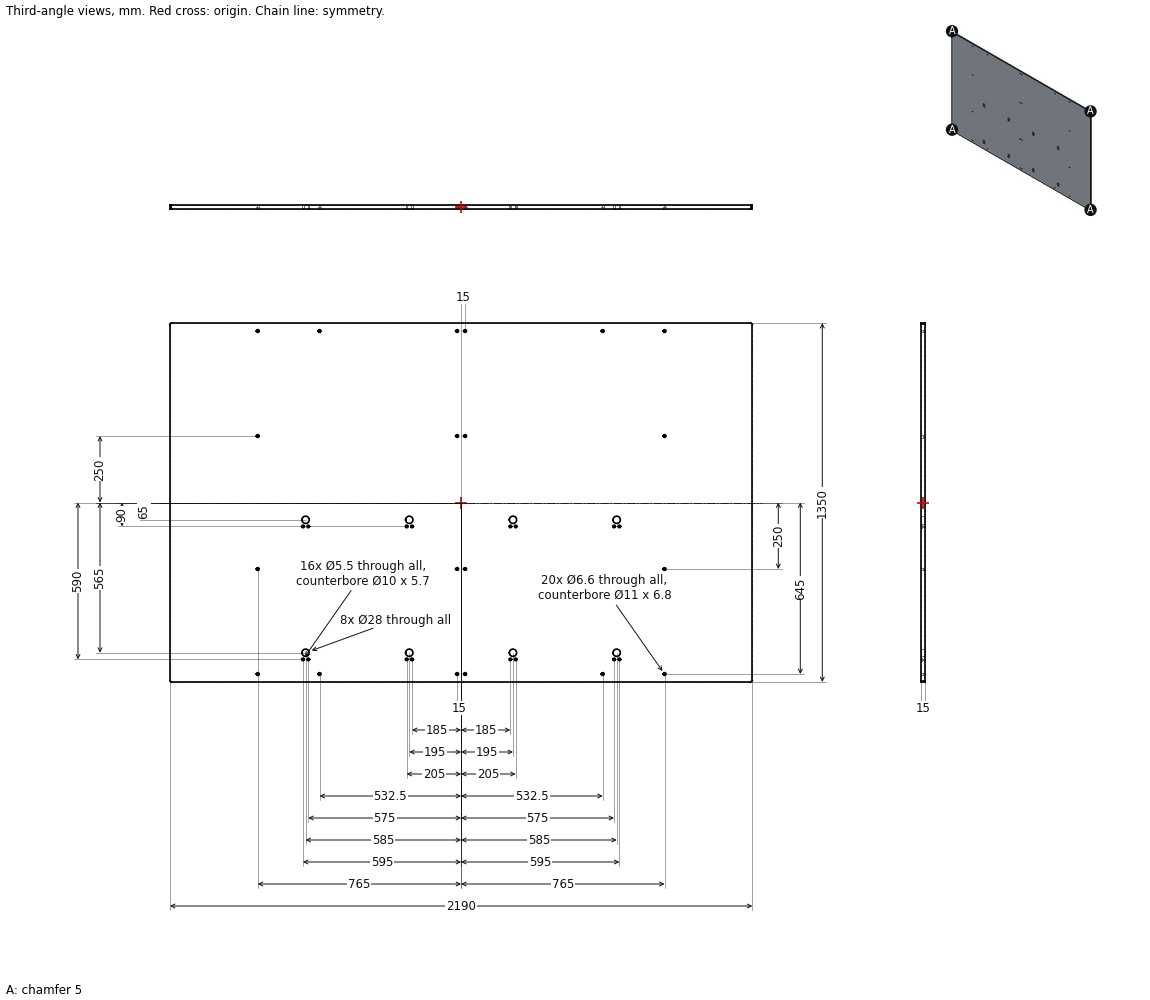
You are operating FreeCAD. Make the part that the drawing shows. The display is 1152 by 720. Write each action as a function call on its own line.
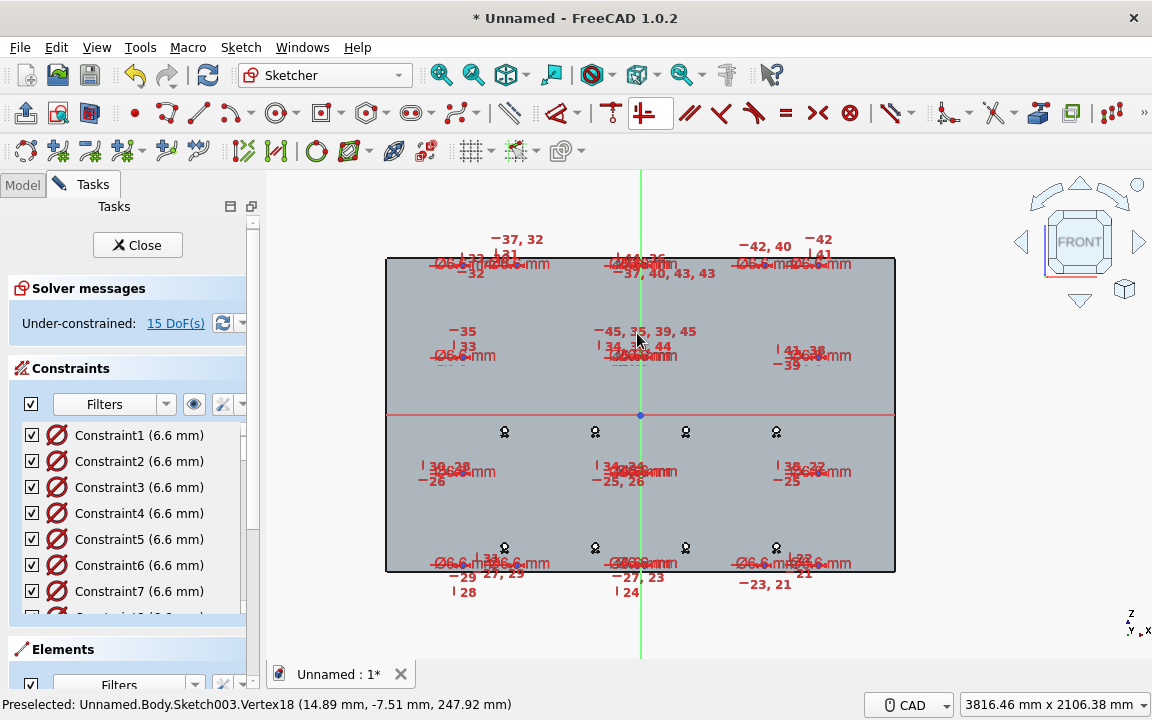
scroll(644, 473, up, 3)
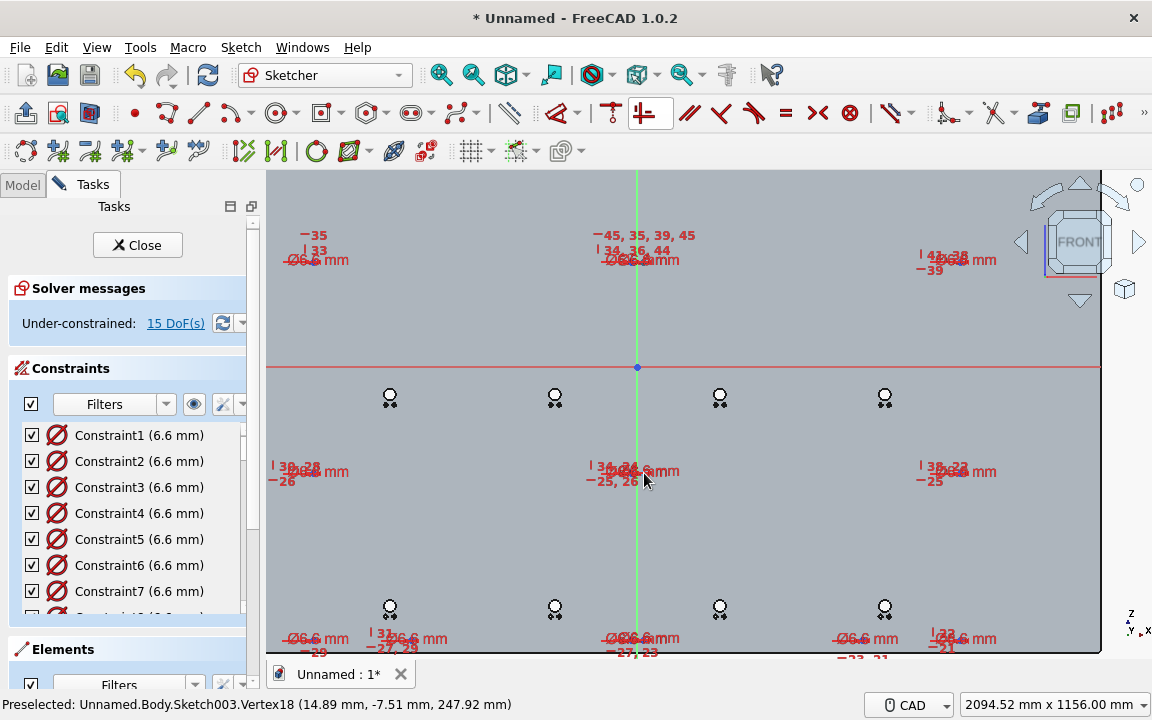
click(644, 473)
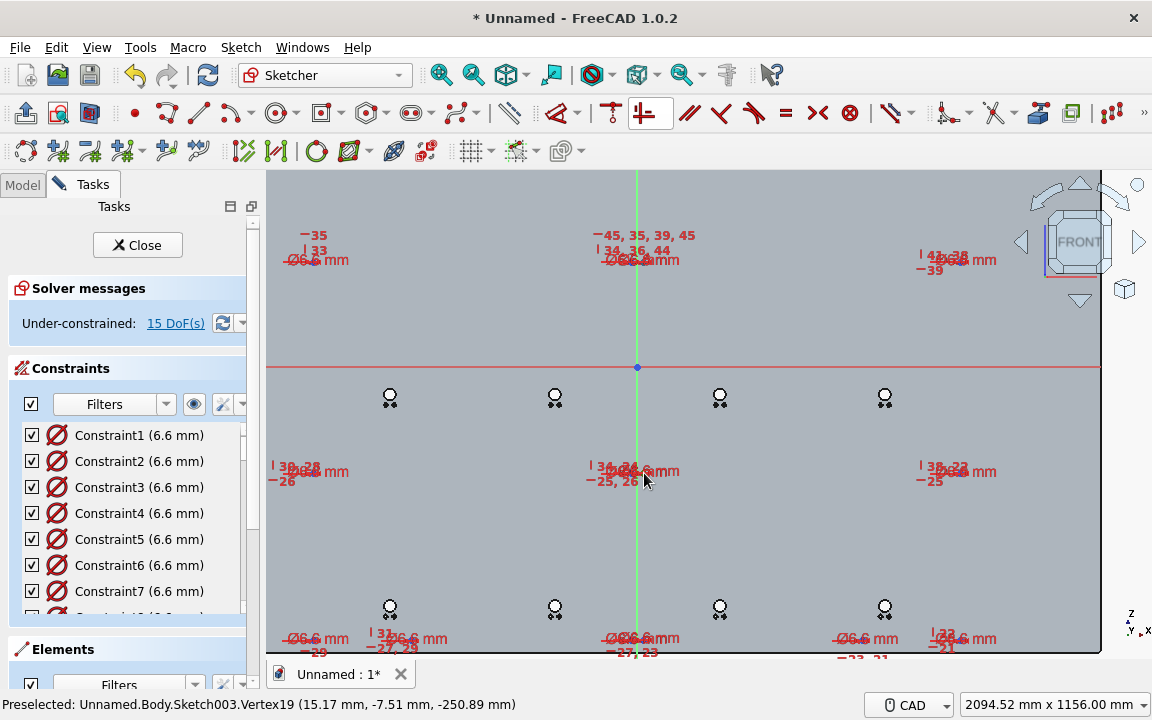
key(v)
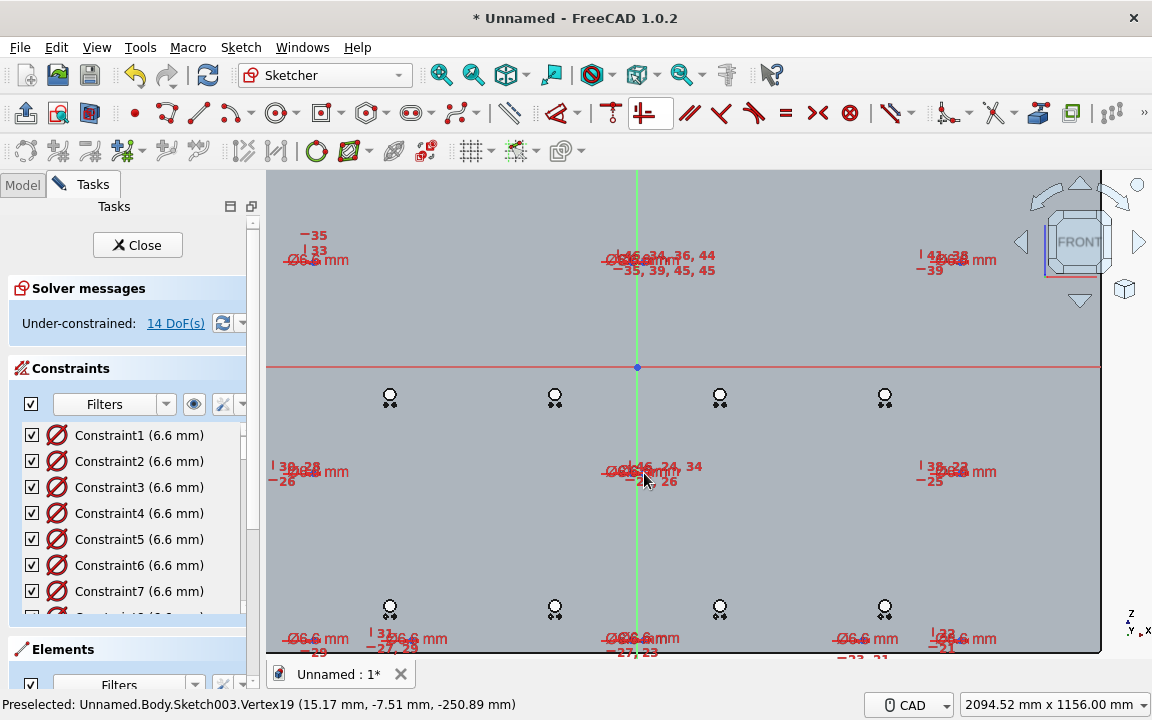
scroll(631, 474, up, 4)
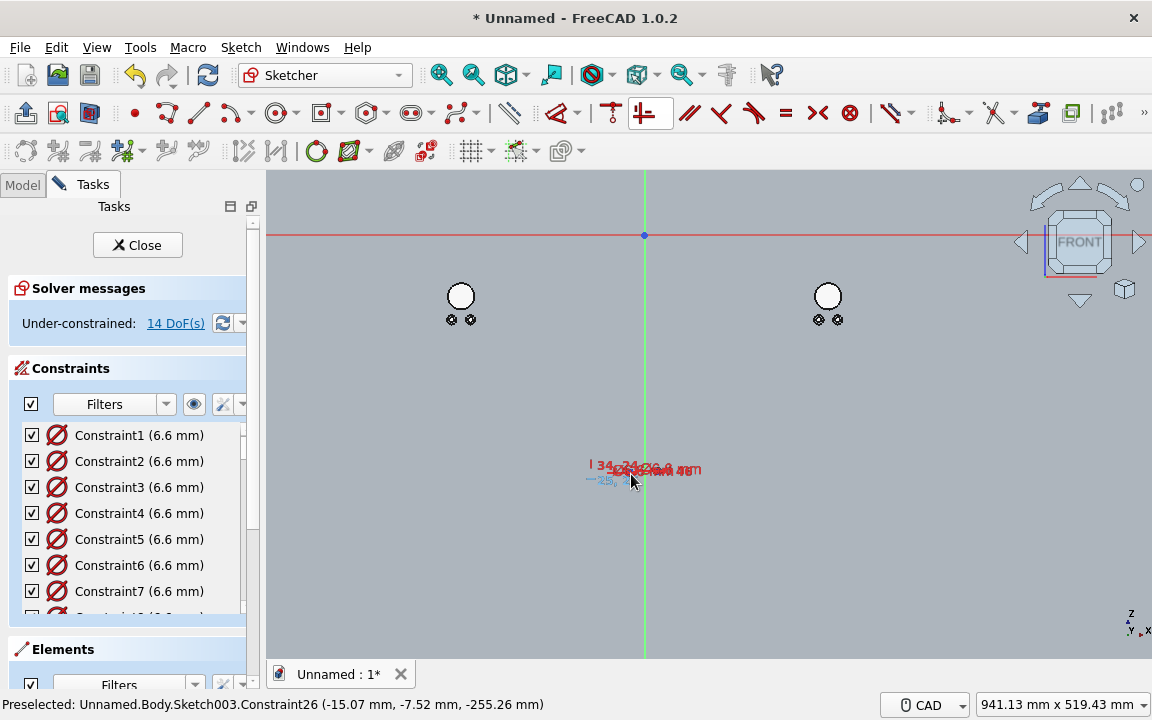
click(631, 473)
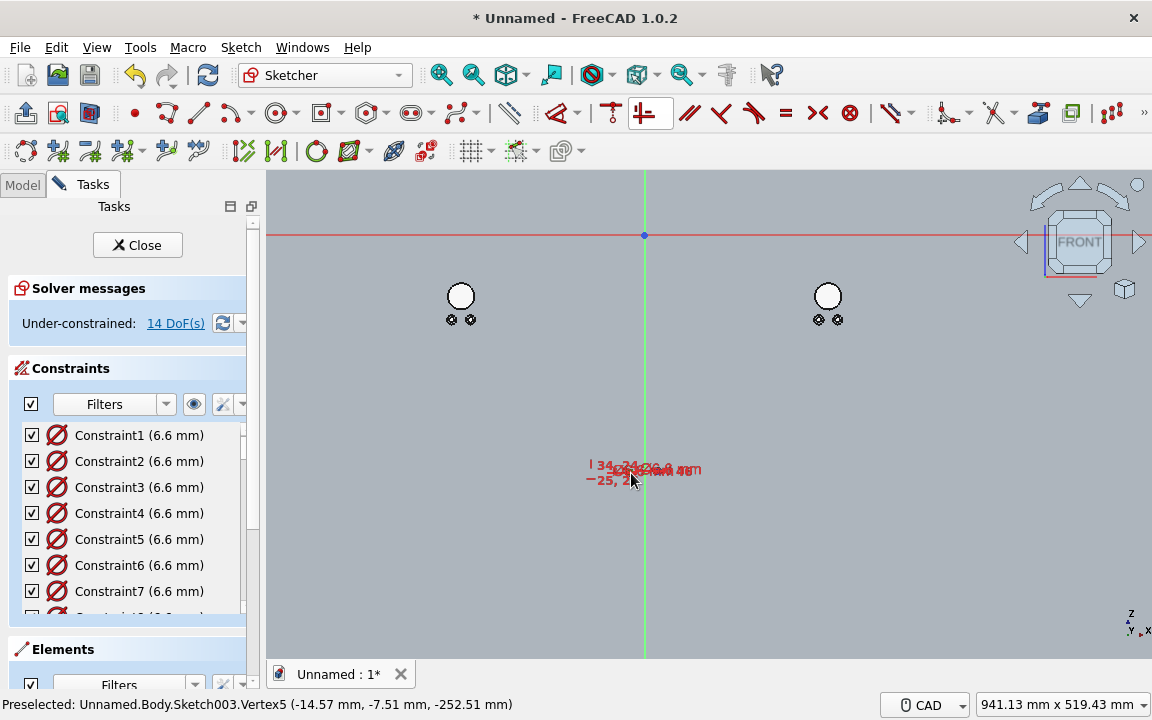
click(659, 471)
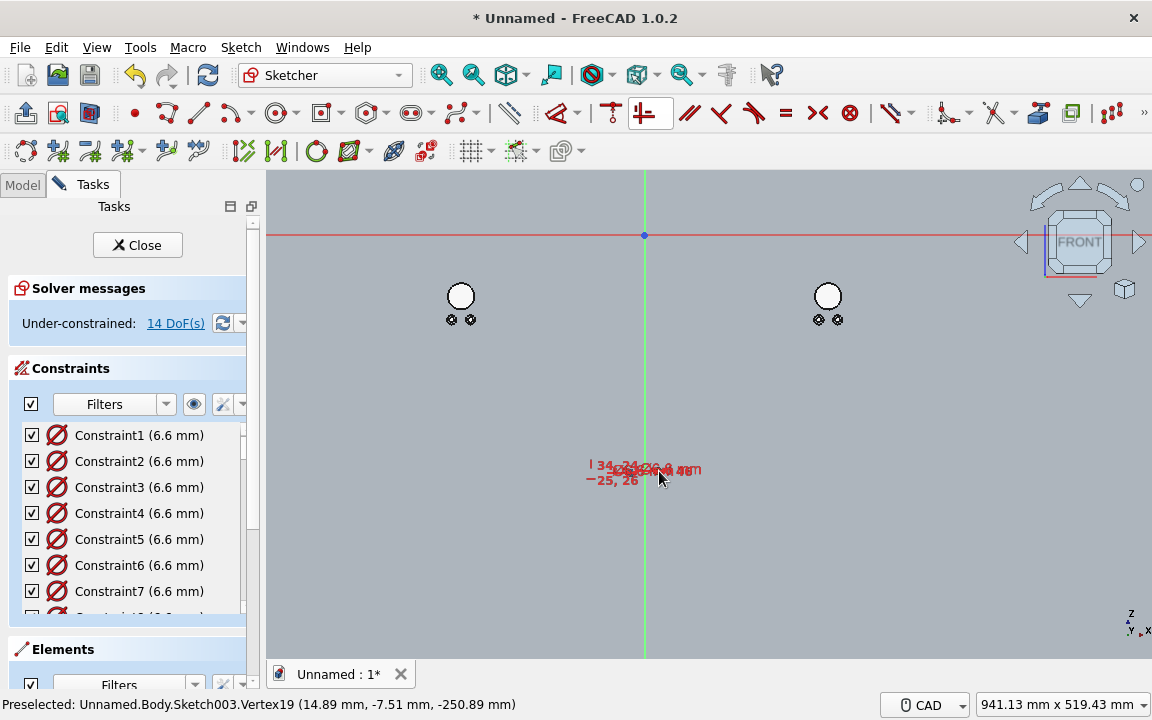
key(h)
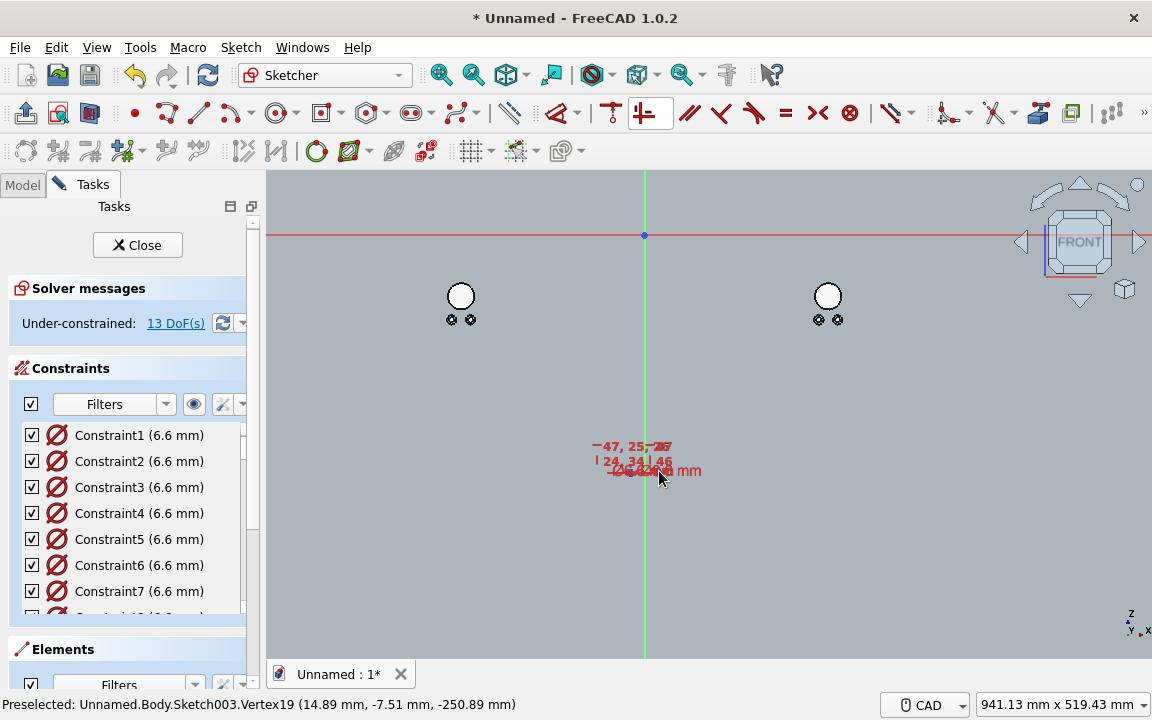
click(659, 473)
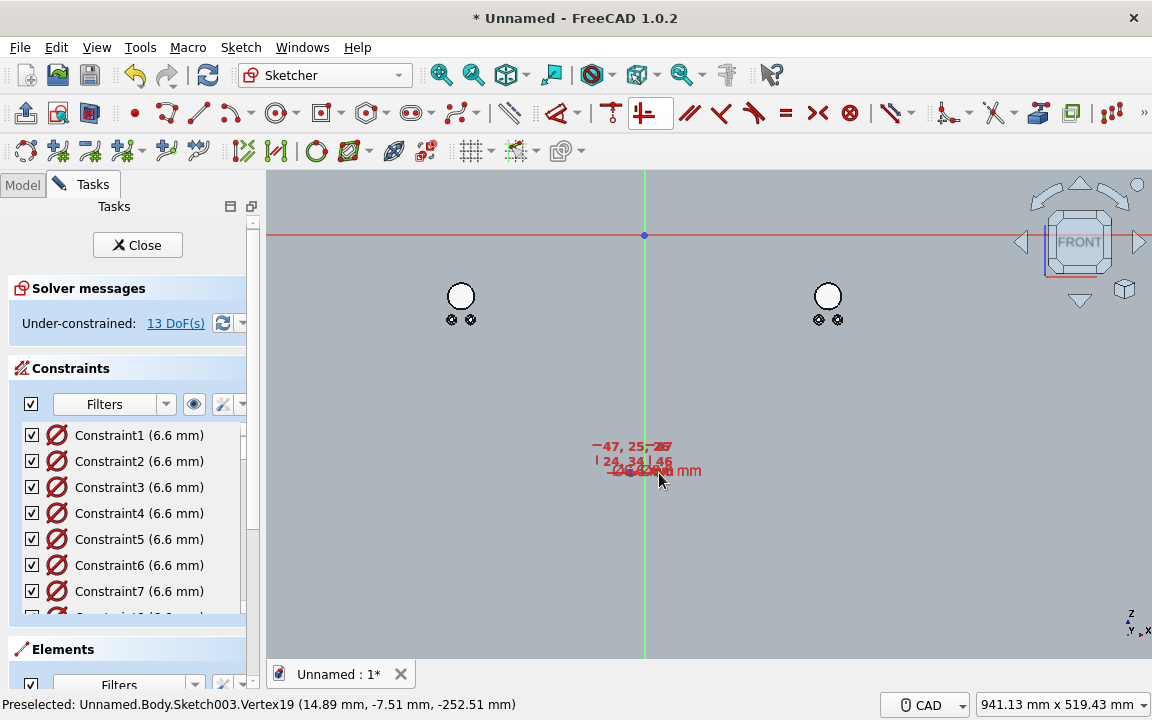
scroll(639, 473, down, 7)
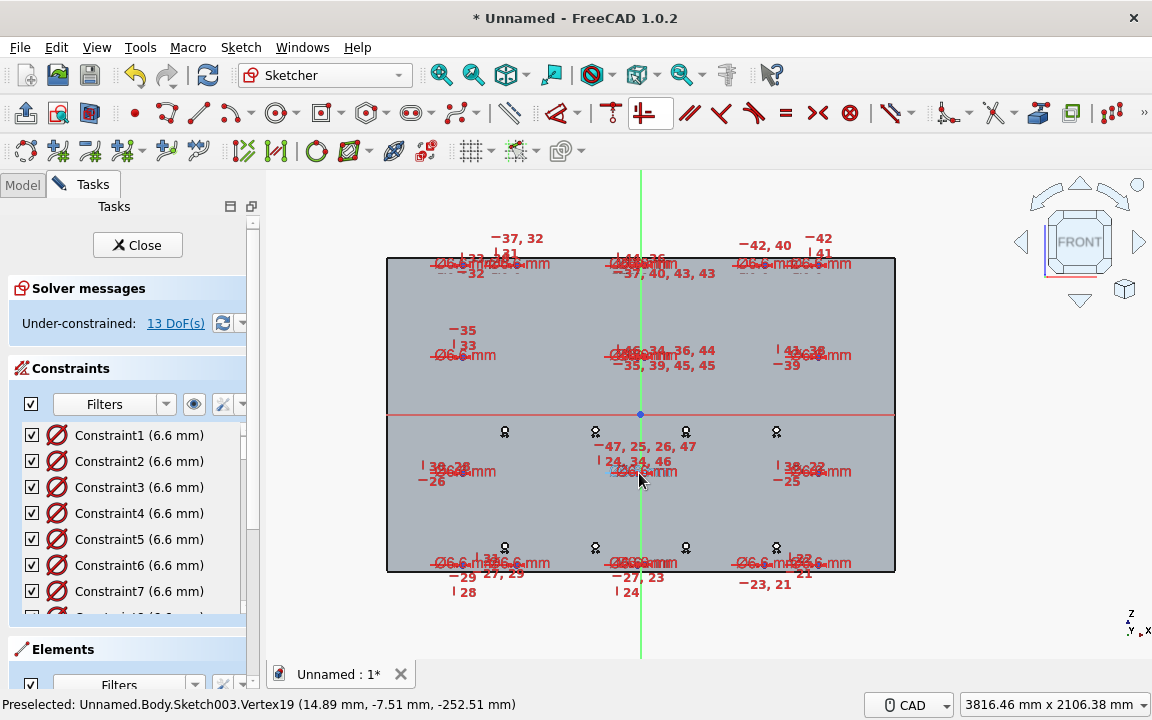
scroll(644, 565, up, 3)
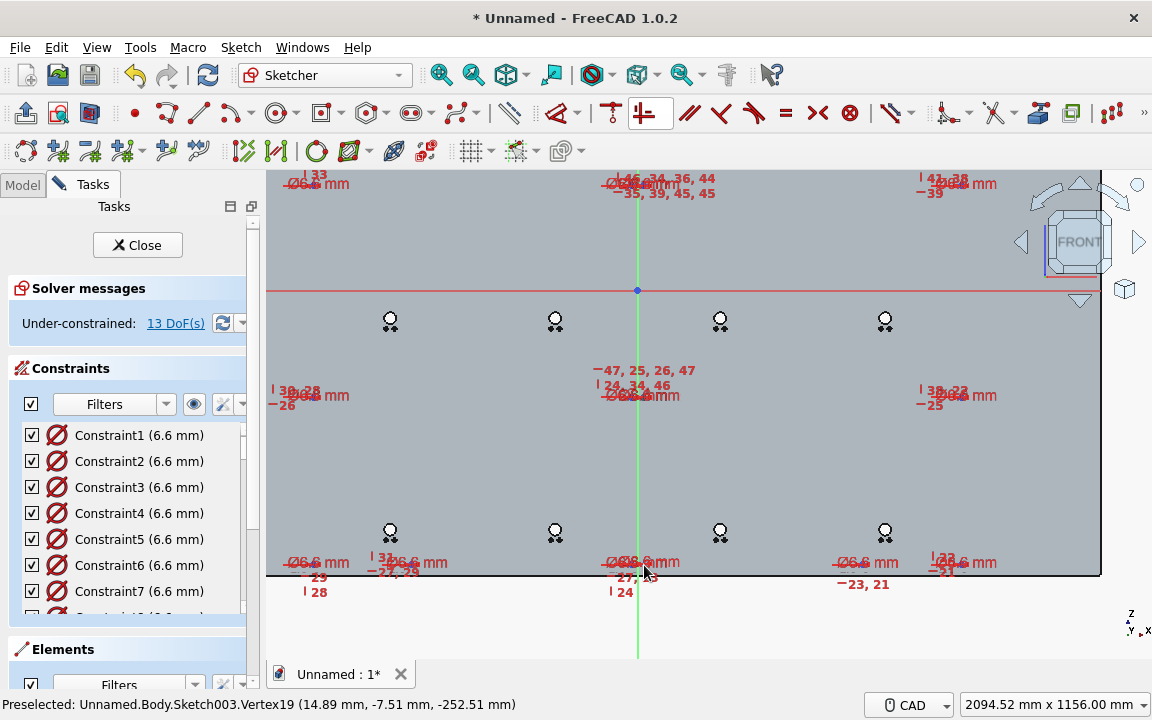
click(644, 564)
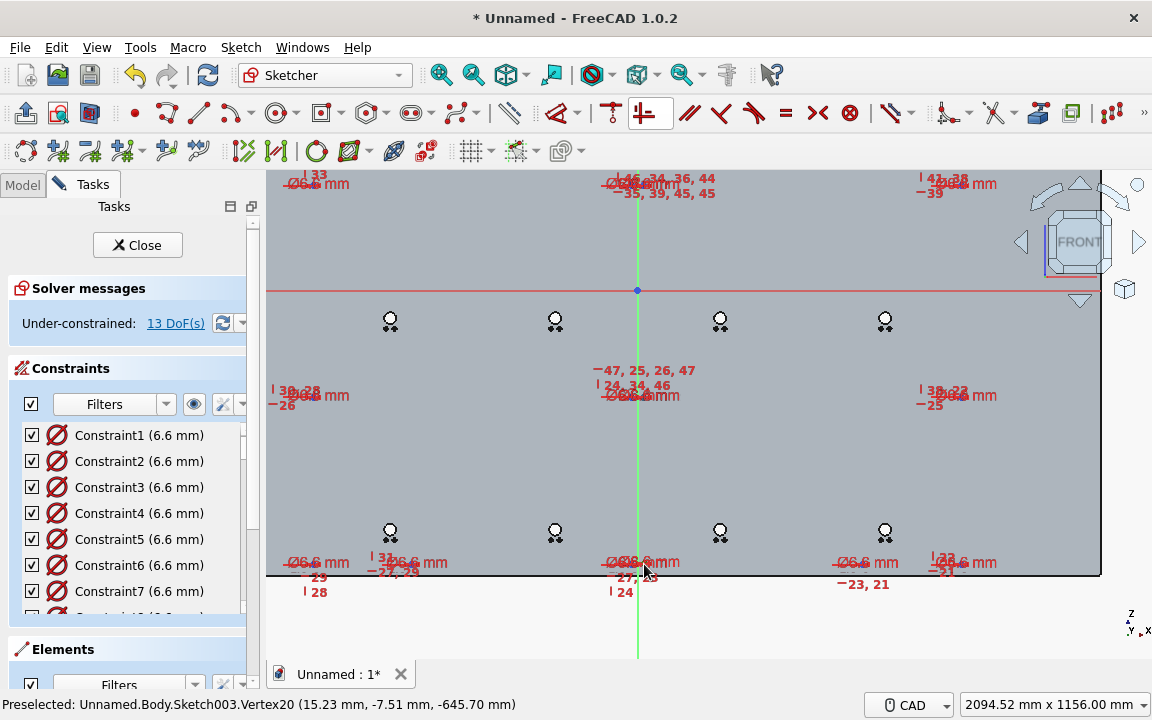
key(v)